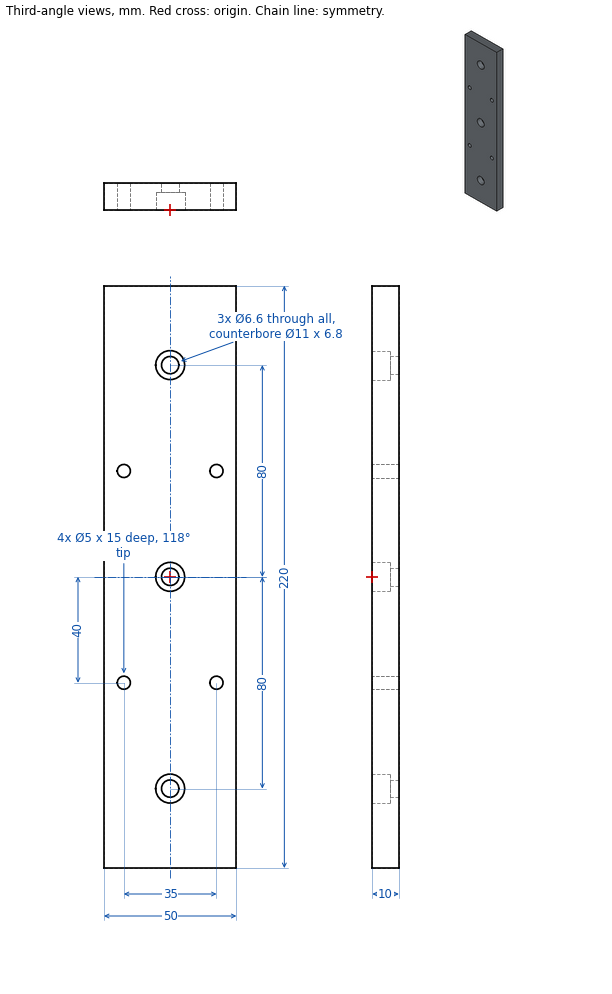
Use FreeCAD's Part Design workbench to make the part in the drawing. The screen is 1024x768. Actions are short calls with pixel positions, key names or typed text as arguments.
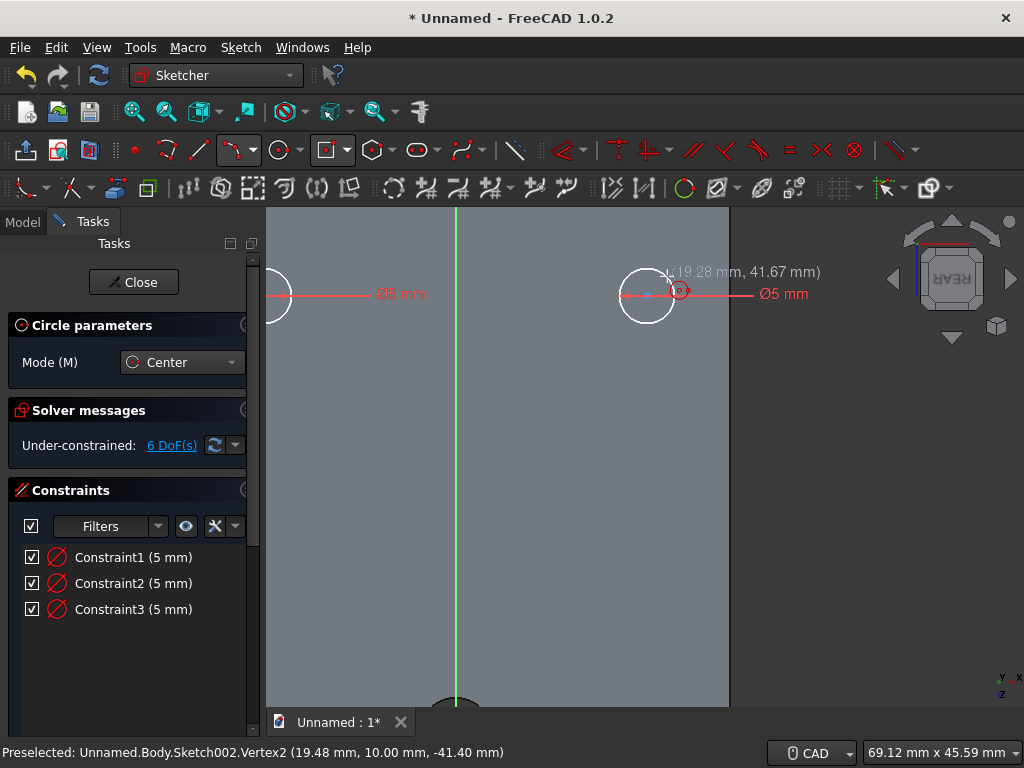
scroll(647, 296, down, 5)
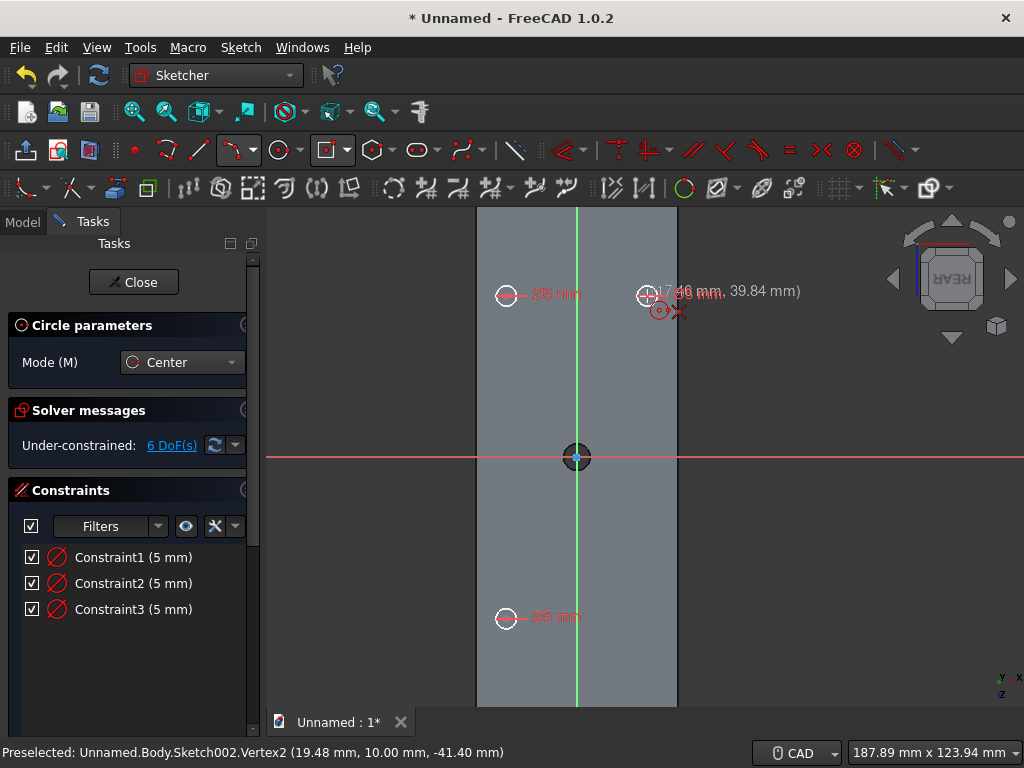
scroll(647, 619, up, 5)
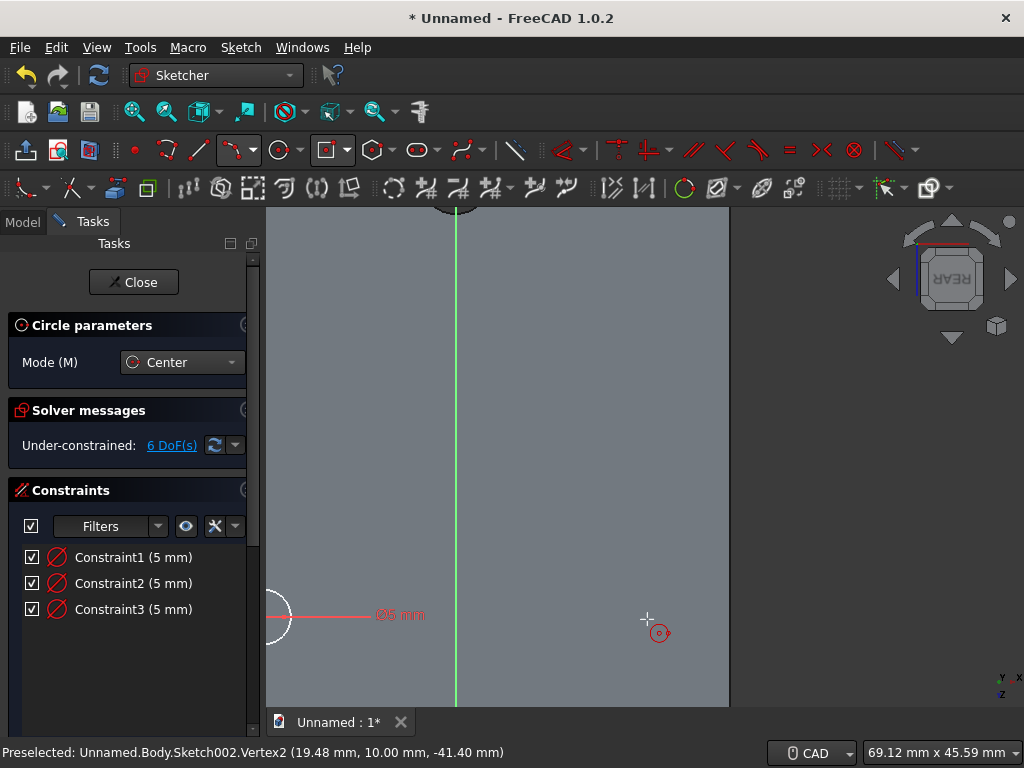
click(647, 616)
move(667, 597)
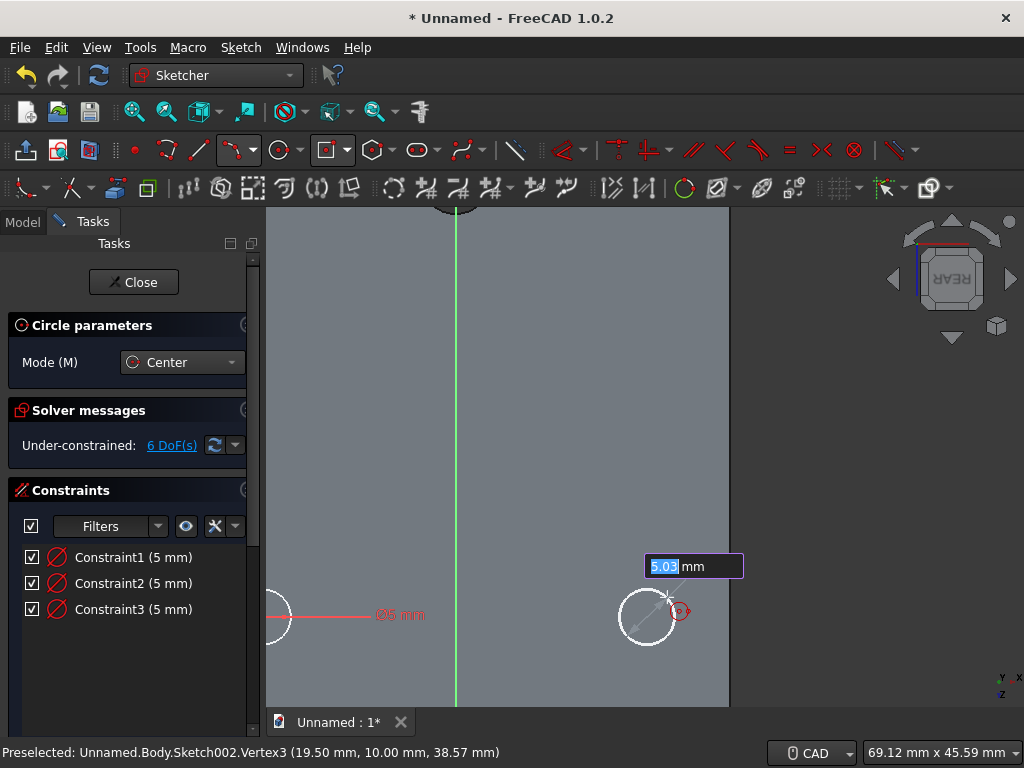
text(5)
key(Return)
key(Escape)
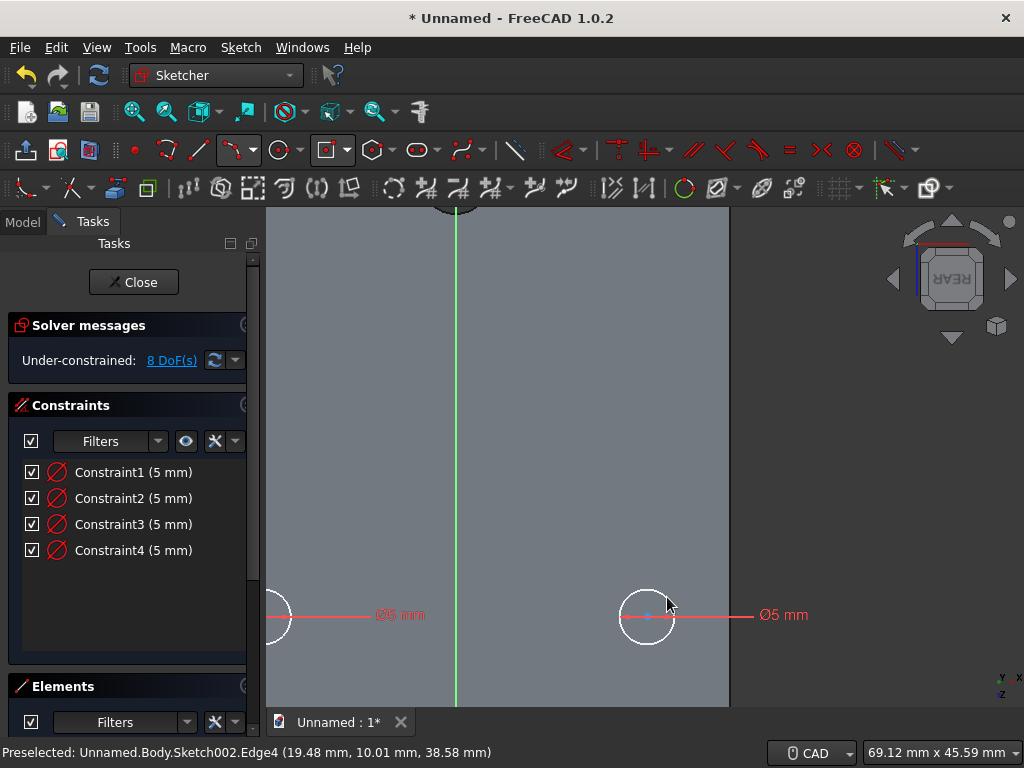
scroll(647, 619, down, 5)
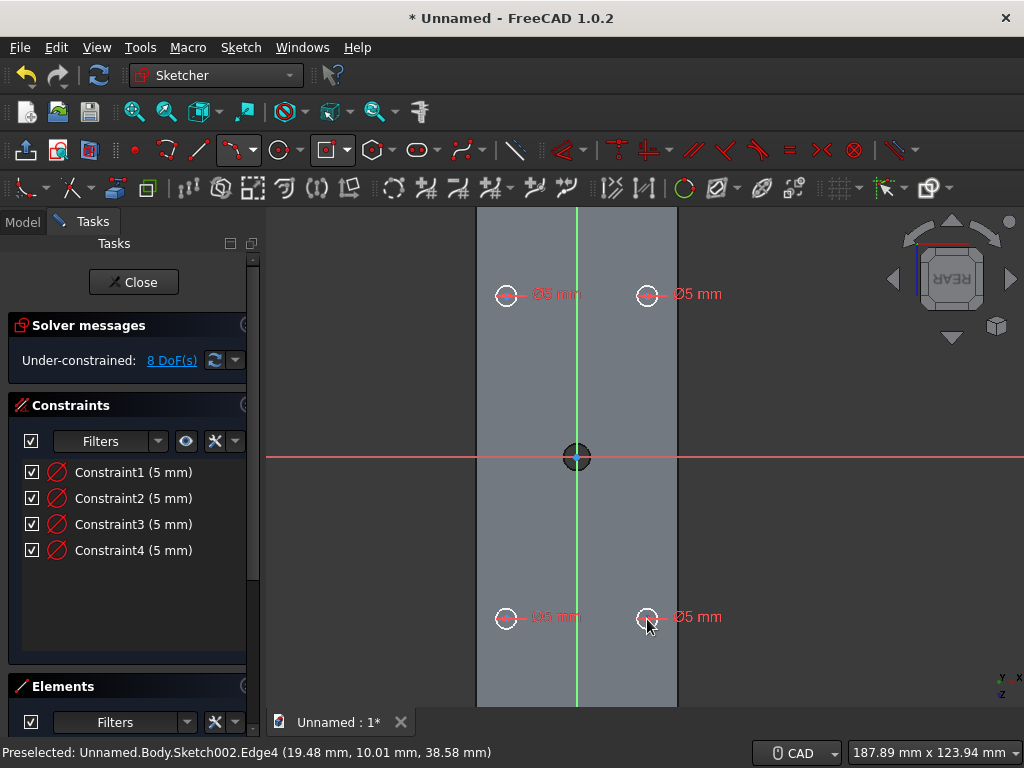
click(506, 296)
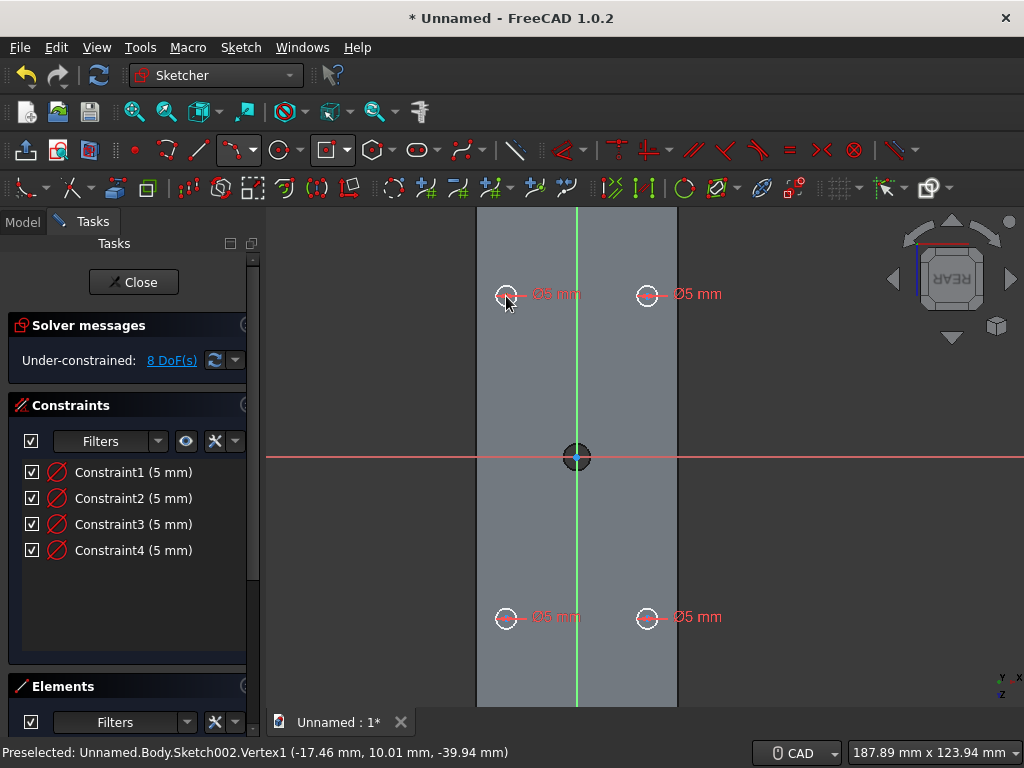
click(506, 619)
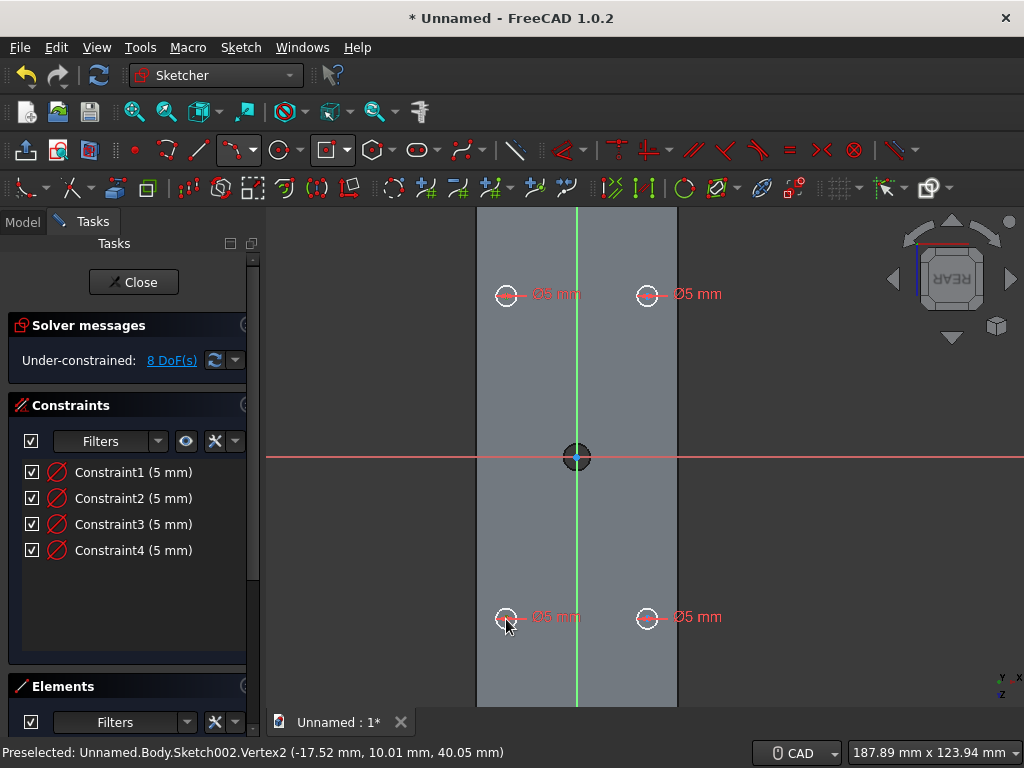
click(334, 457)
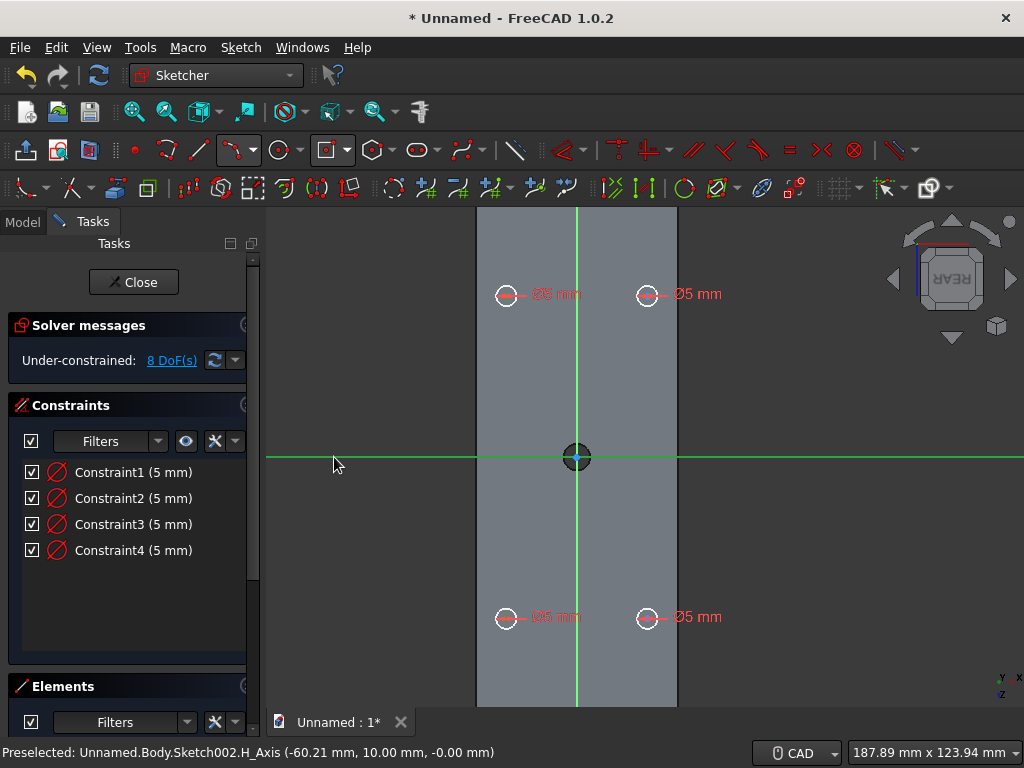
click(822, 150)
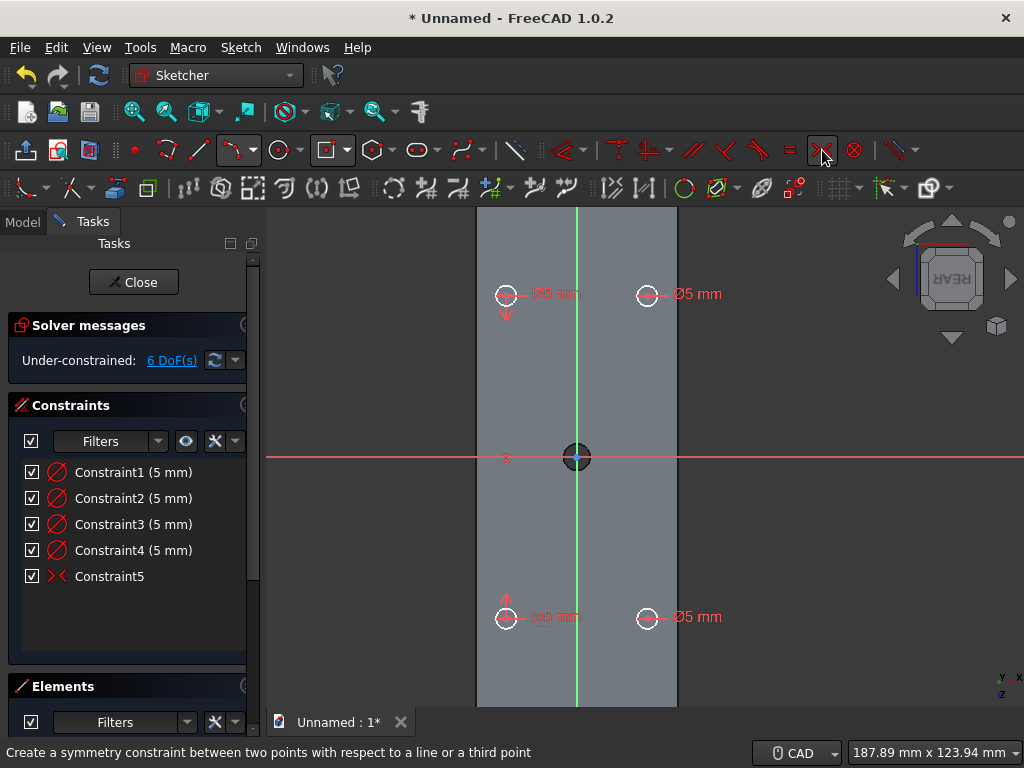
click(506, 296)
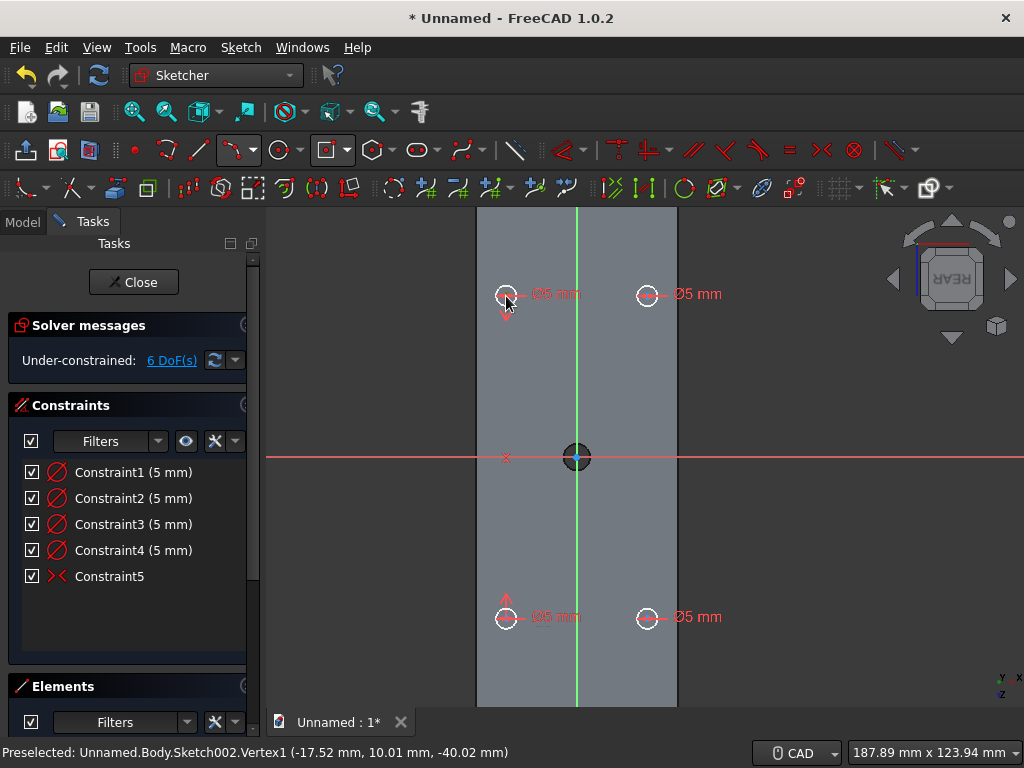
click(647, 296)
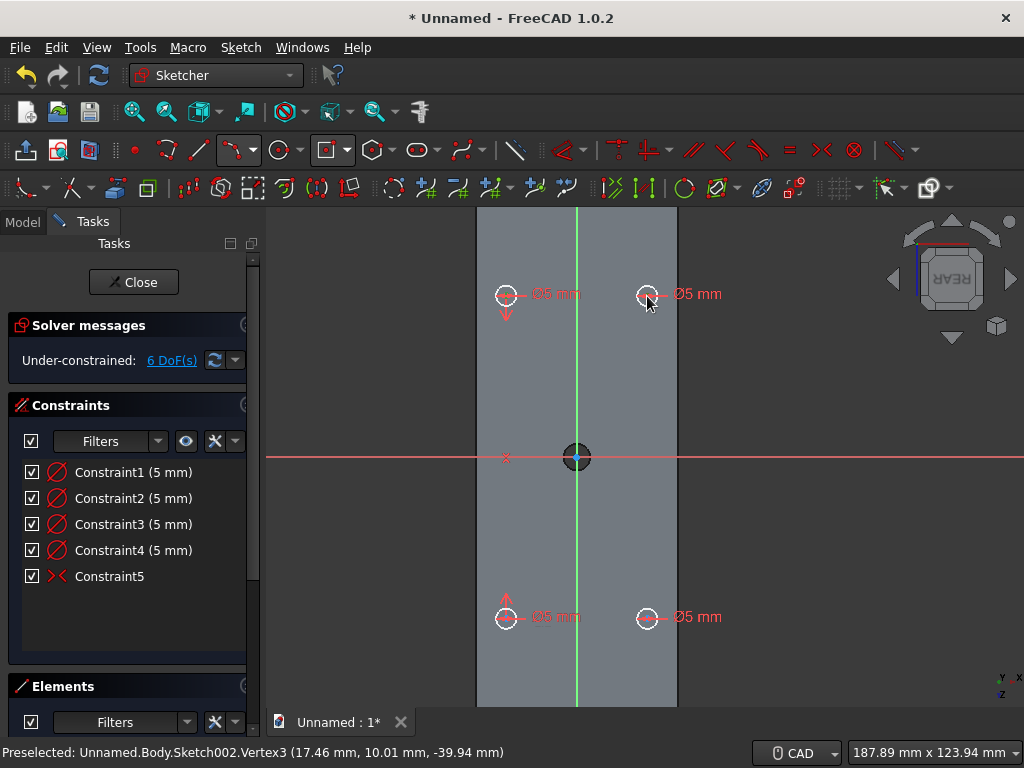
click(577, 647)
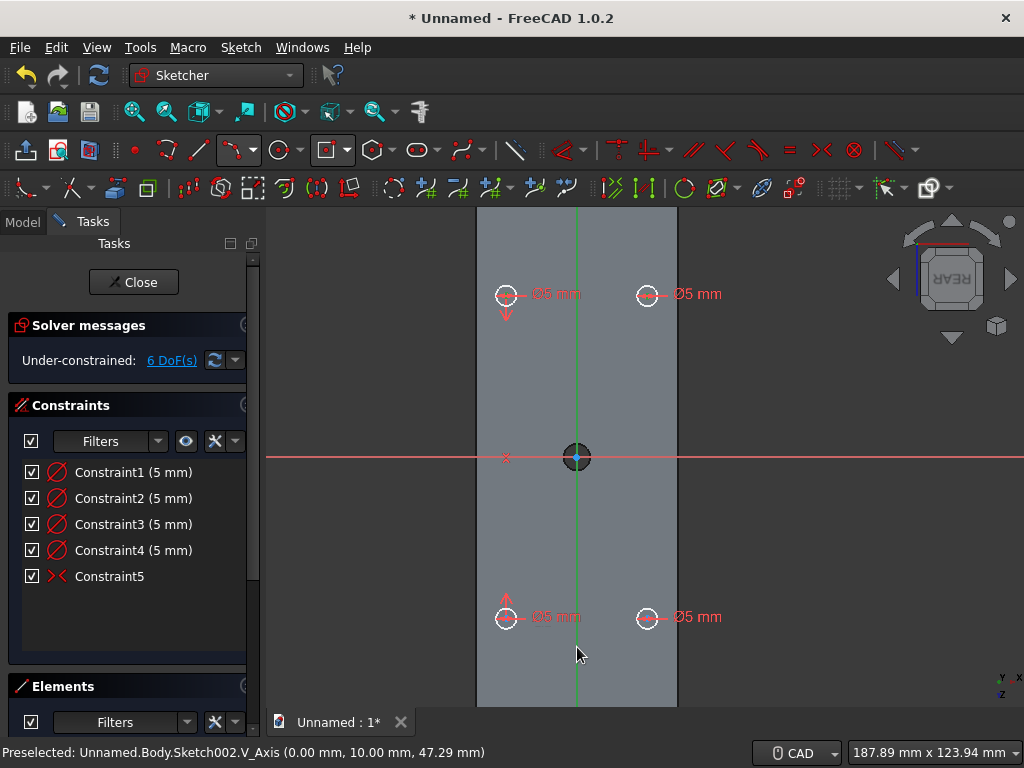
click(822, 150)